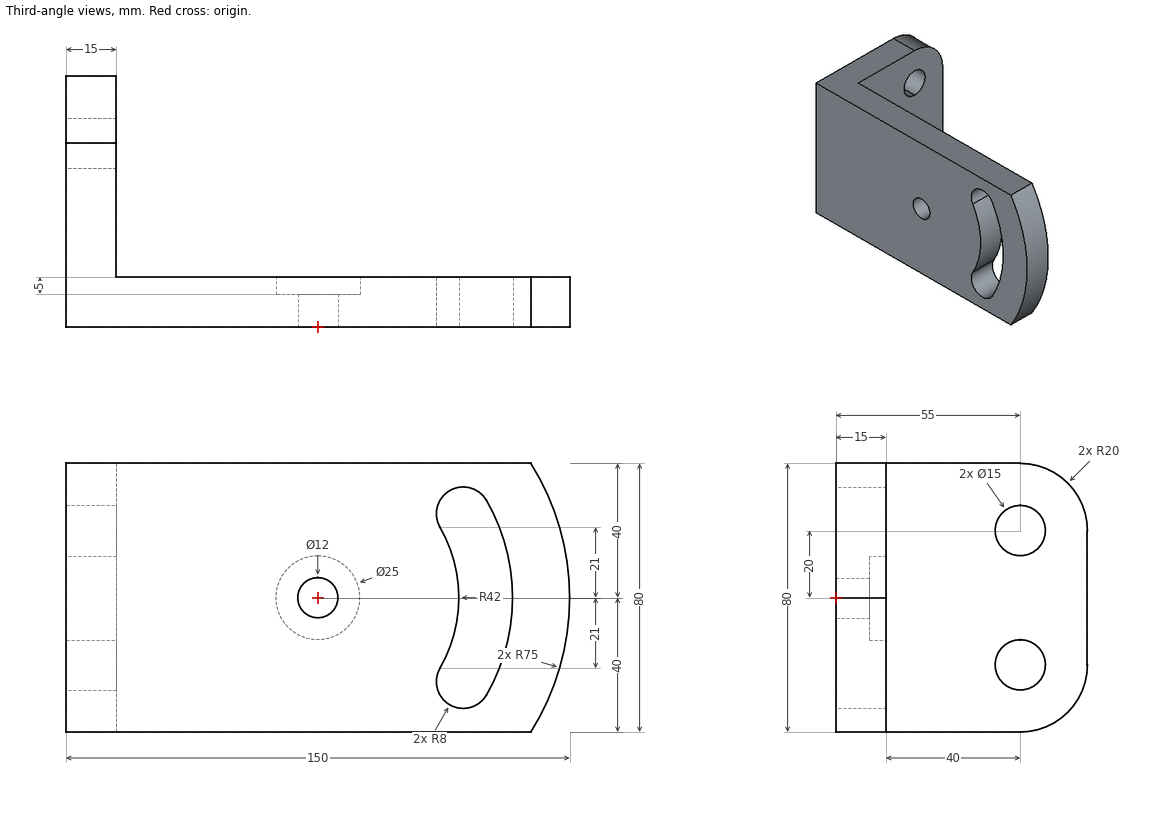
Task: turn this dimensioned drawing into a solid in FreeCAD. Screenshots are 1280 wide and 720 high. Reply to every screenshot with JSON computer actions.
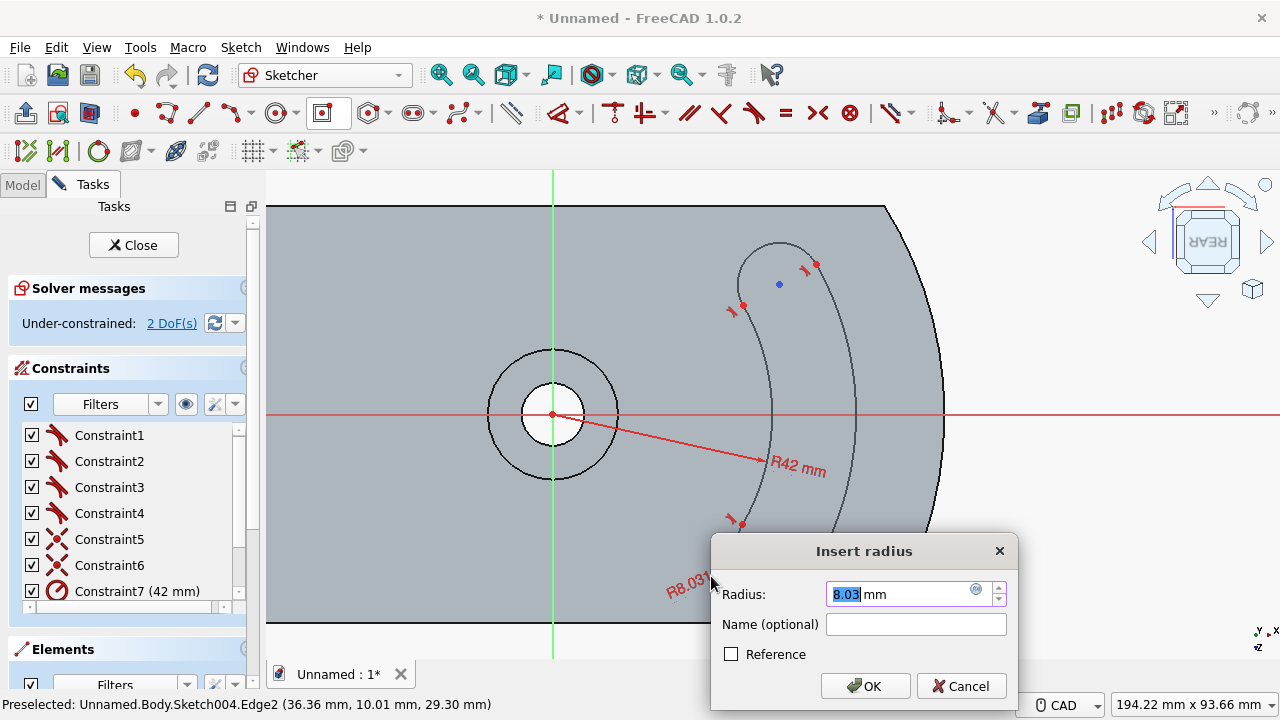
{"action": "type", "text": "8"}
{"action": "key", "text": "Return"}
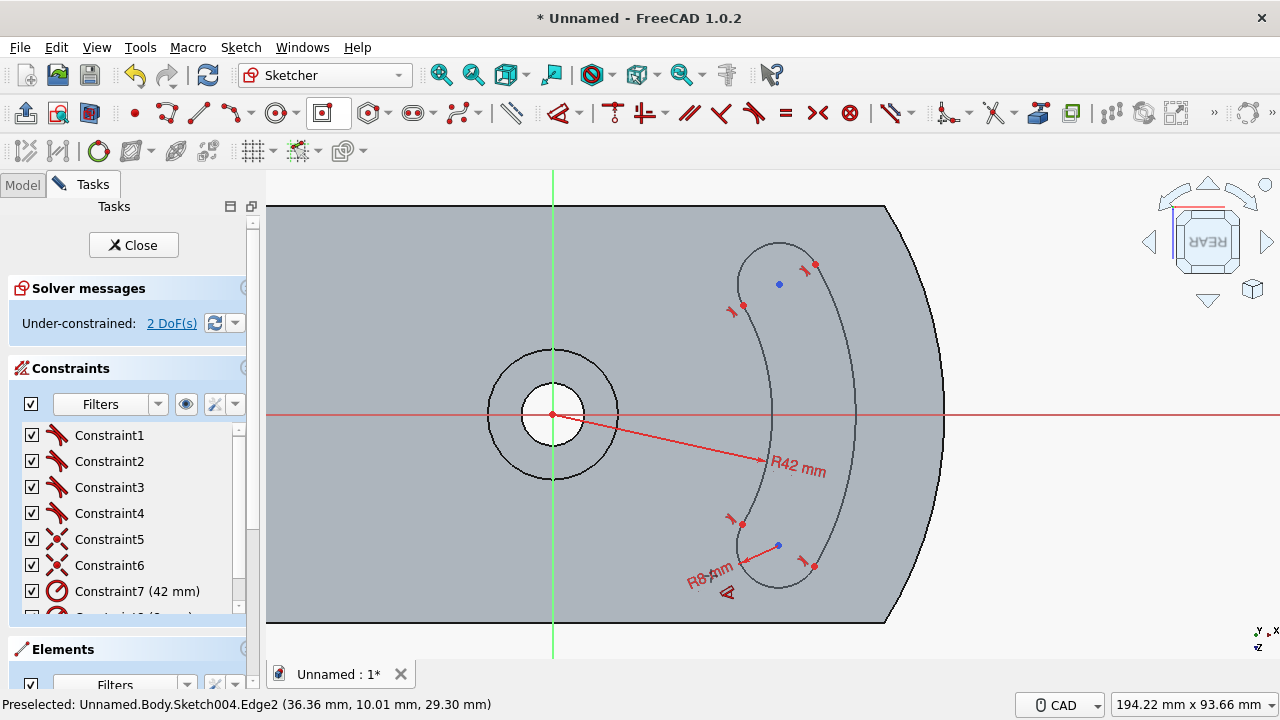
{"action": "left_click", "coordinate": [742, 525]}
{"action": "left_click", "coordinate": [519, 470]}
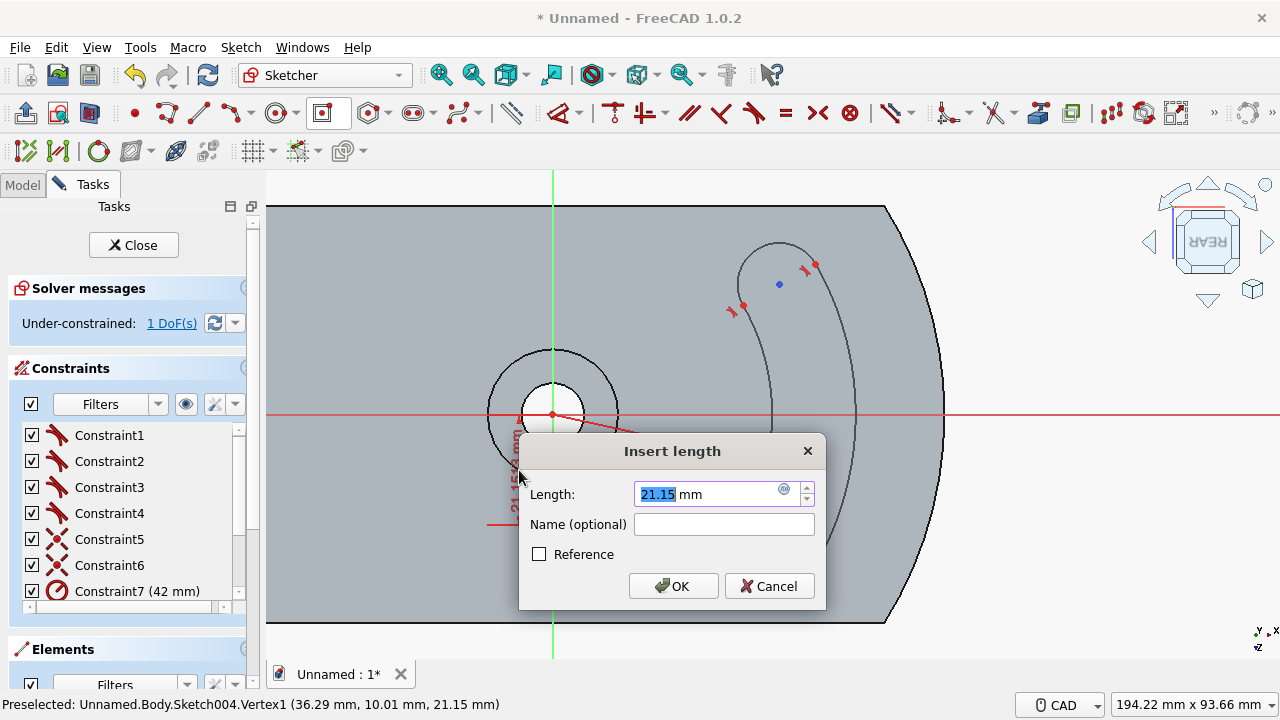
{"action": "type", "text": "21"}
{"action": "key", "text": "Return"}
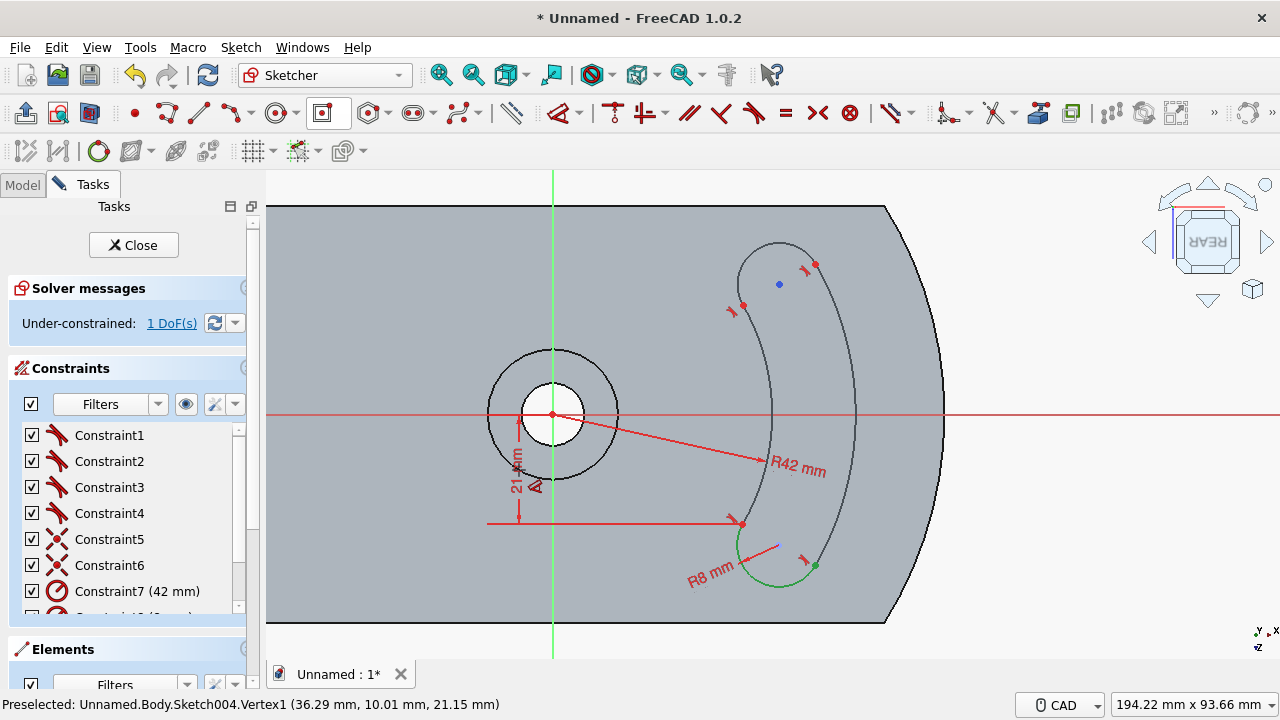
{"action": "left_click", "coordinate": [743, 306]}
{"action": "left_click", "coordinate": [519, 360]}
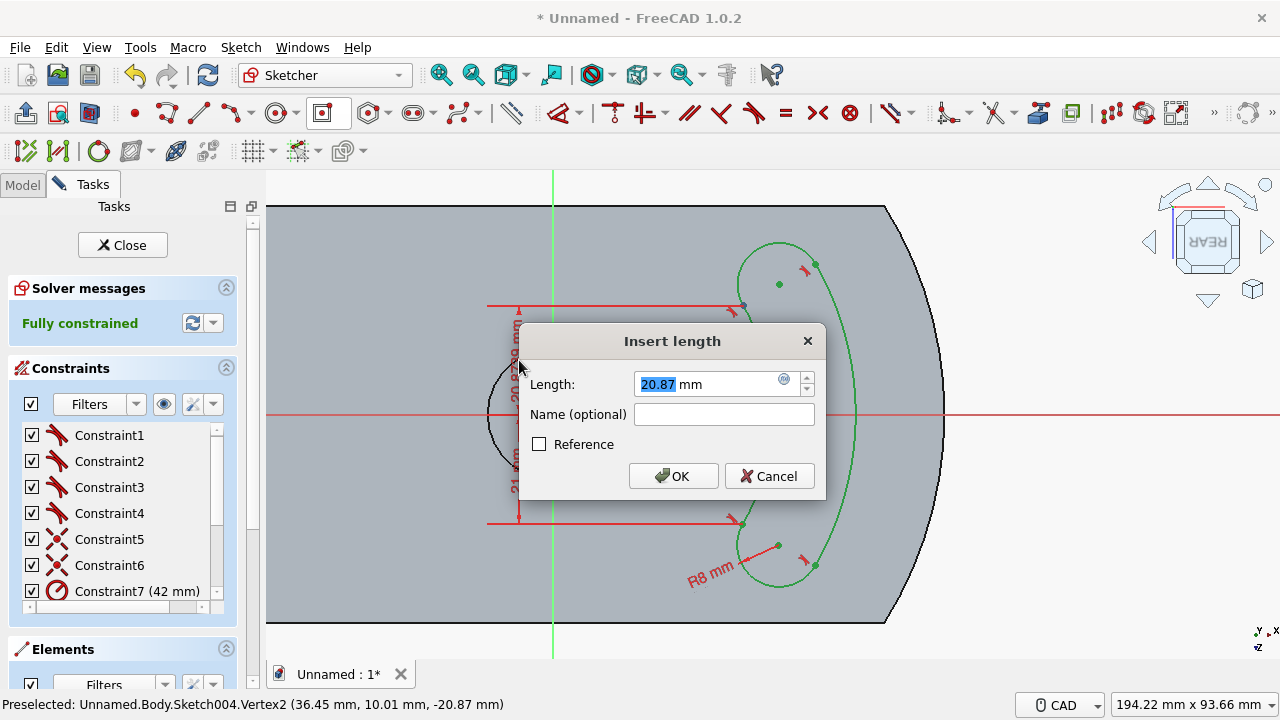
{"action": "type", "text": "21"}
{"action": "key", "text": "Return"}
{"action": "key", "text": "Escape"}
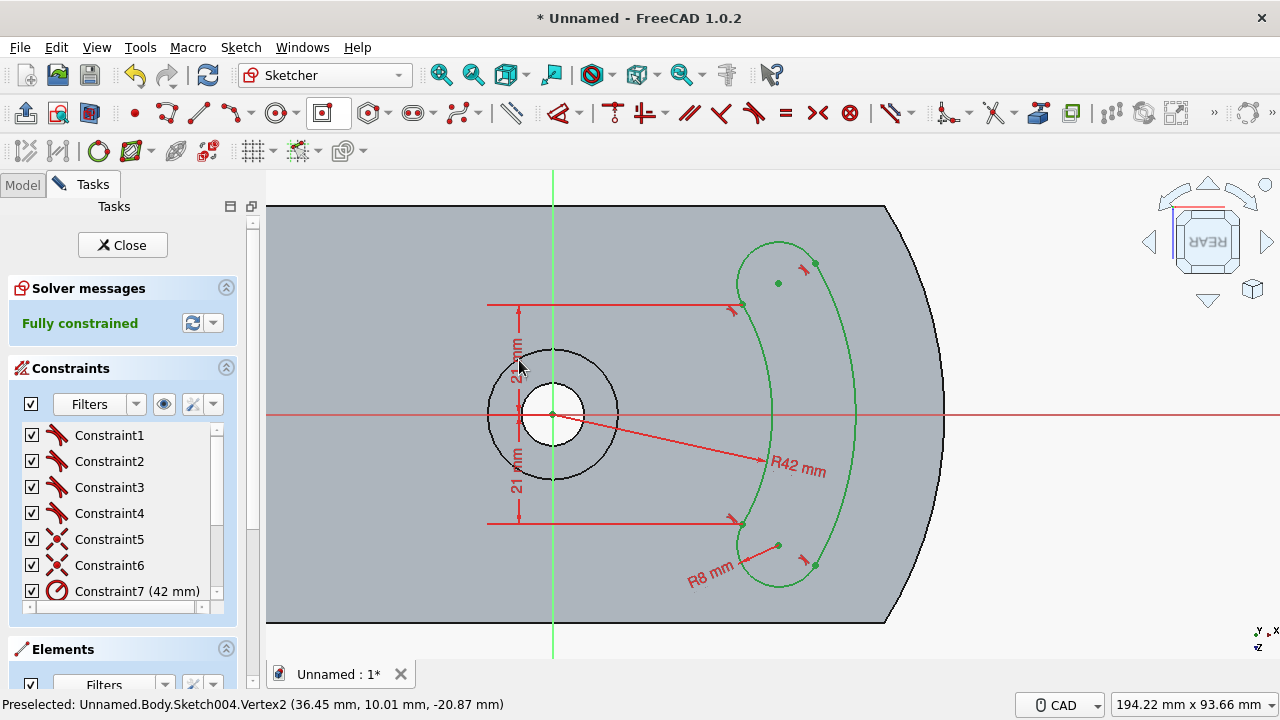
{"action": "left_click", "coordinate": [123, 245]}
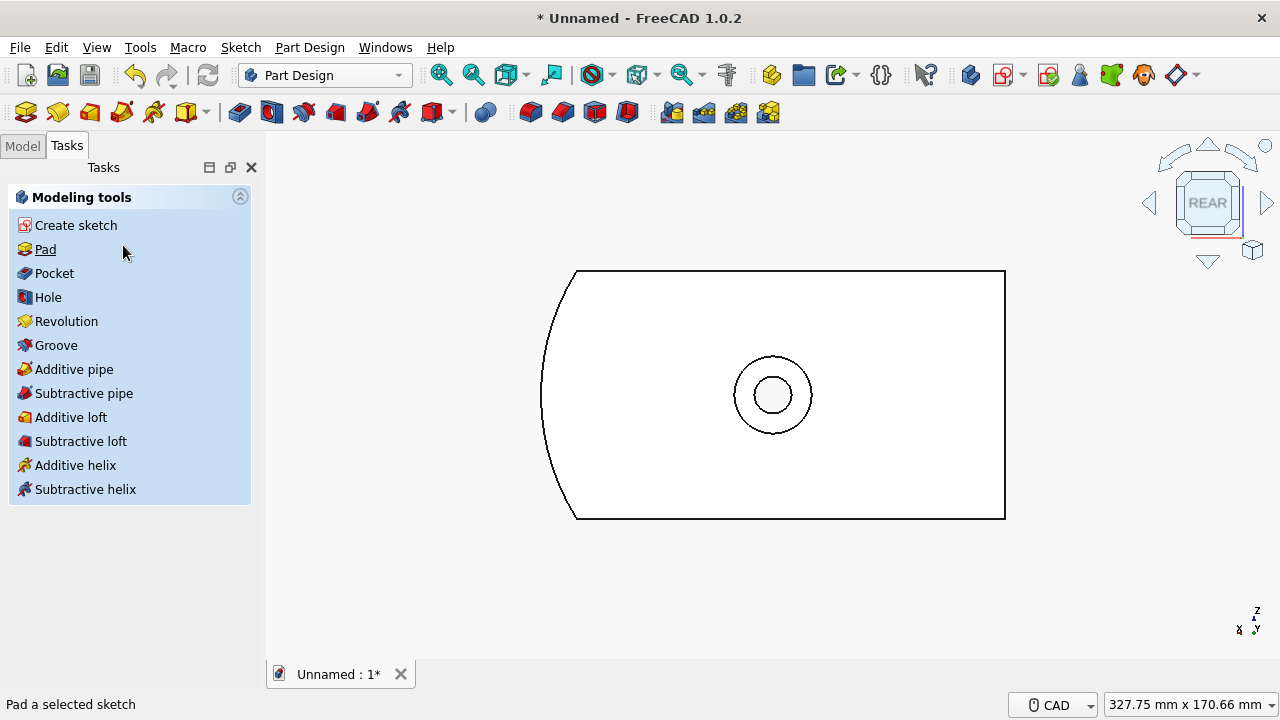
{"action": "left_click", "coordinate": [240, 112]}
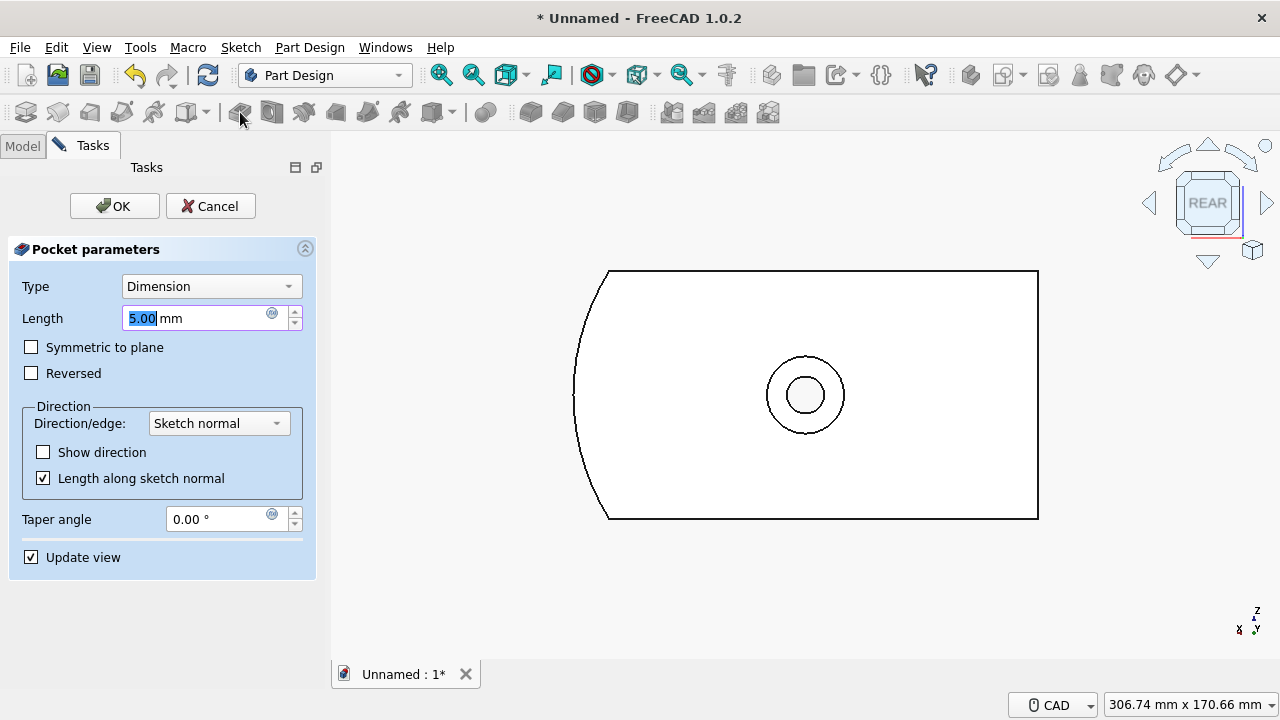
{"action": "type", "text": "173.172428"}
{"action": "key", "text": "Tab"}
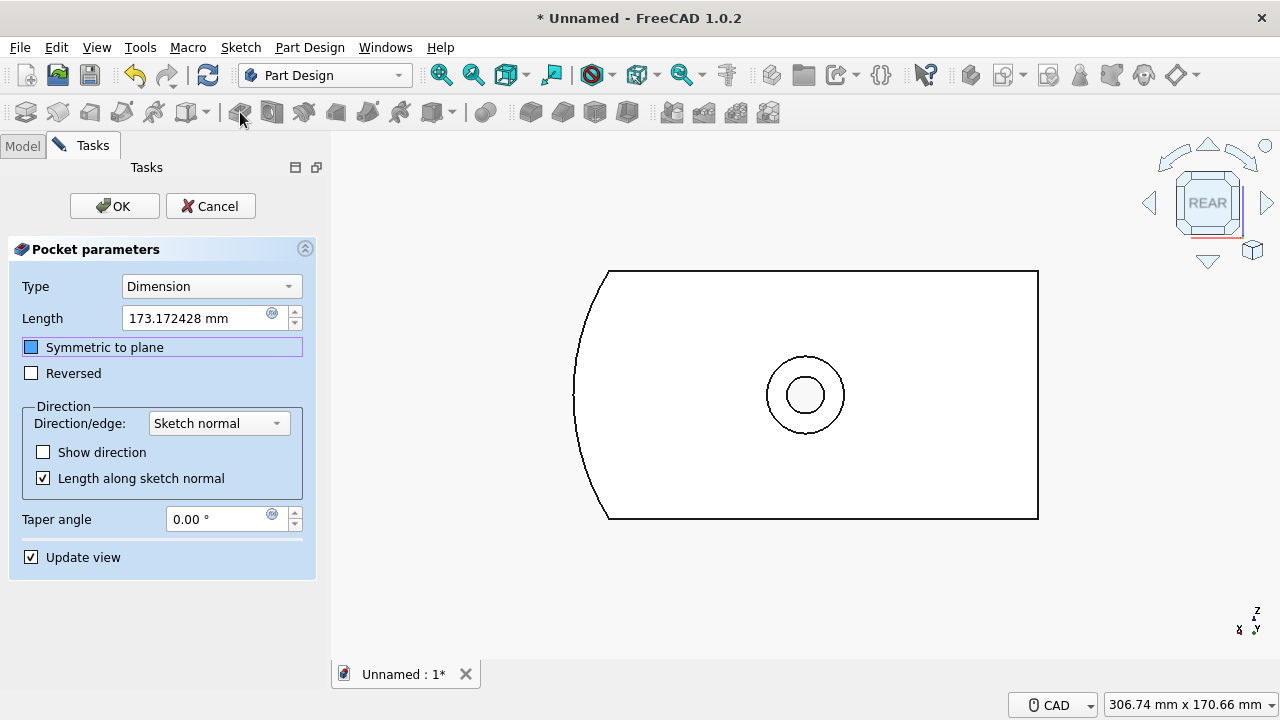
{"action": "left_click", "coordinate": [30, 347]}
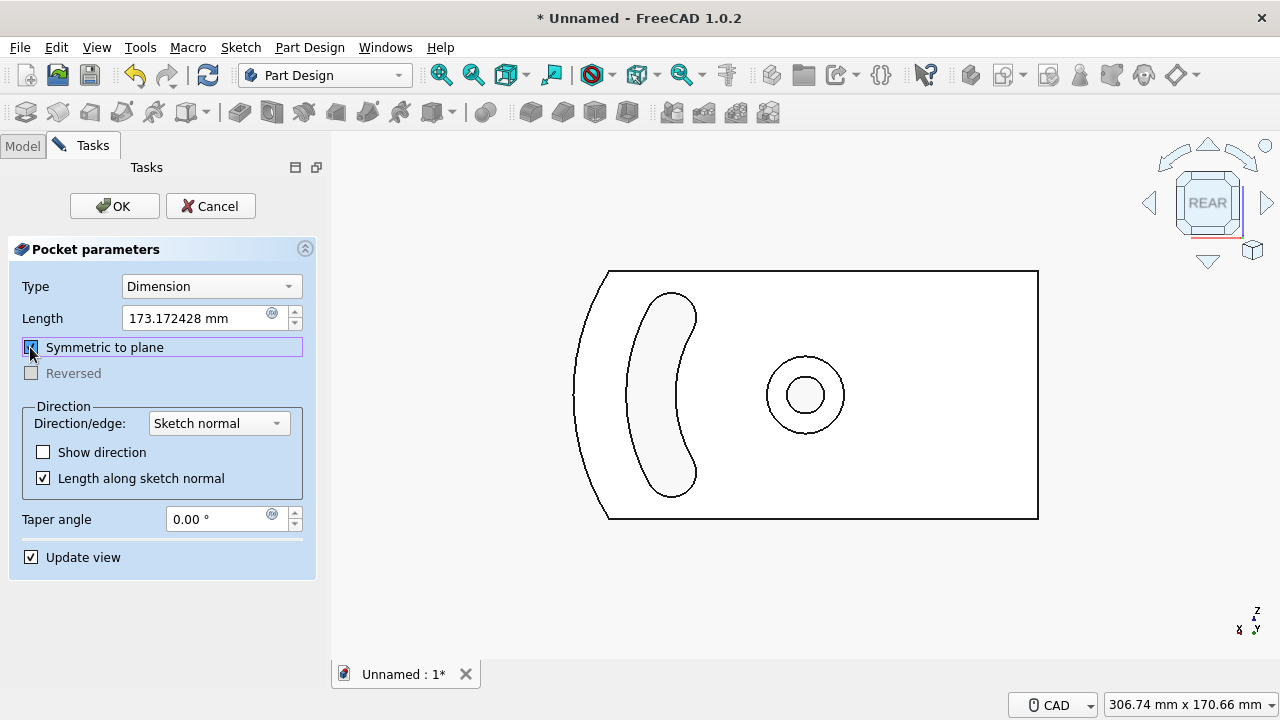
{"action": "left_click", "coordinate": [115, 206]}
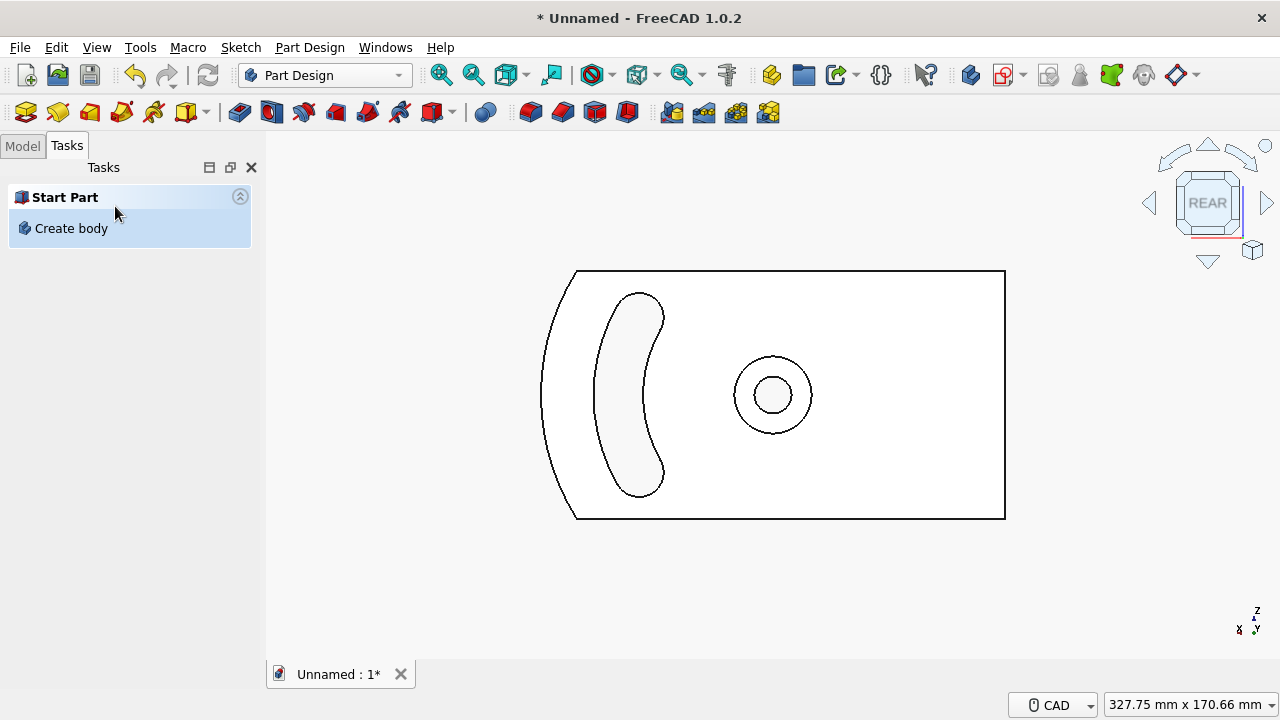
{"action": "key", "text": "6"}